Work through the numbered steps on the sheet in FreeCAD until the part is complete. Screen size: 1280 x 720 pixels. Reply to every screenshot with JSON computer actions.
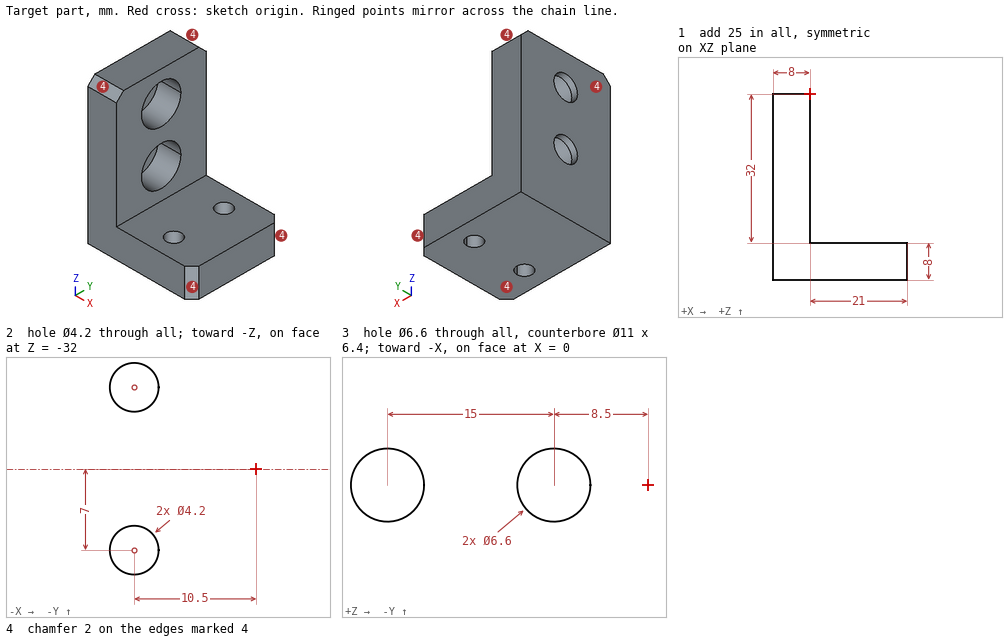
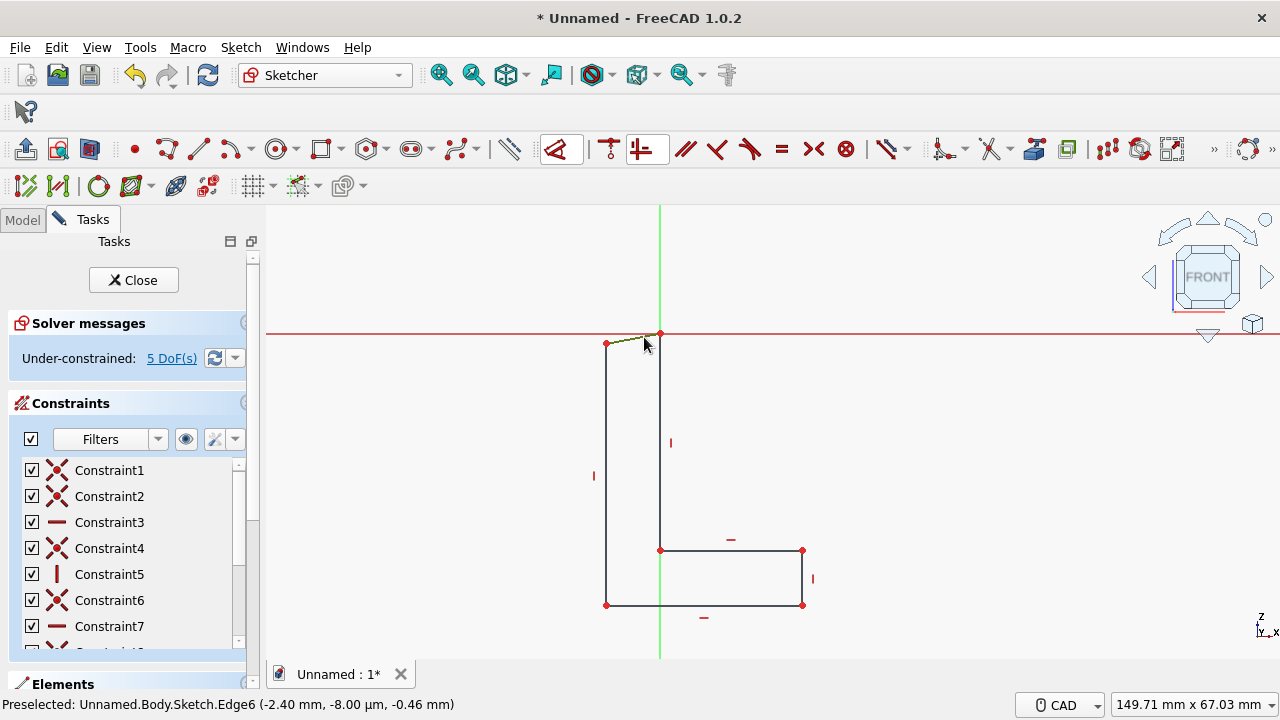
{"action": "left_click", "coordinate": [664, 150]}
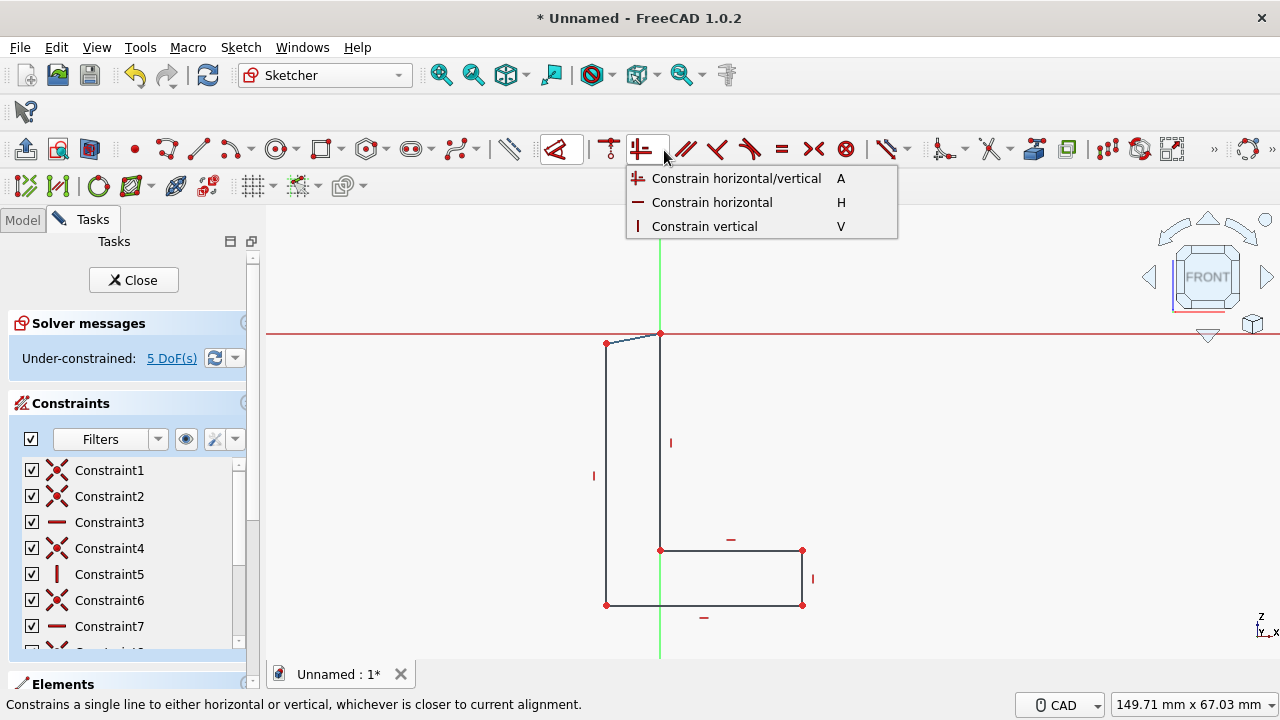
{"action": "left_click", "coordinate": [762, 202]}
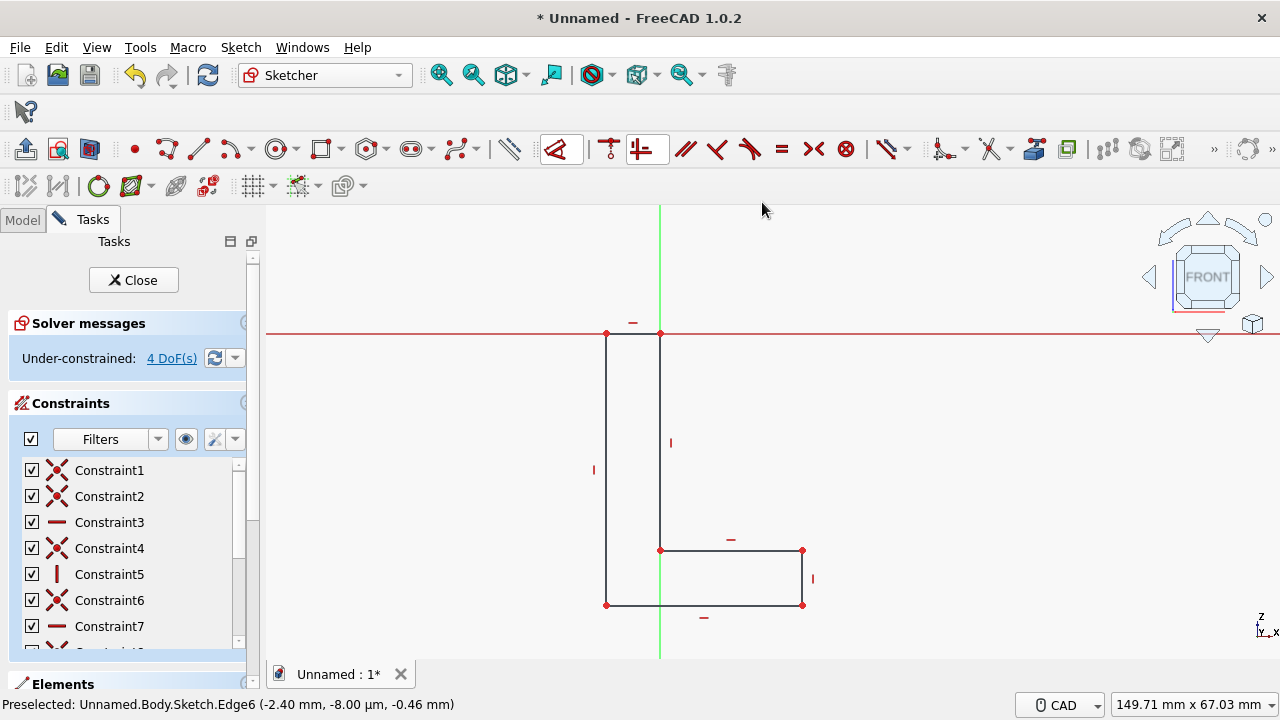
{"action": "left_click", "coordinate": [556, 150]}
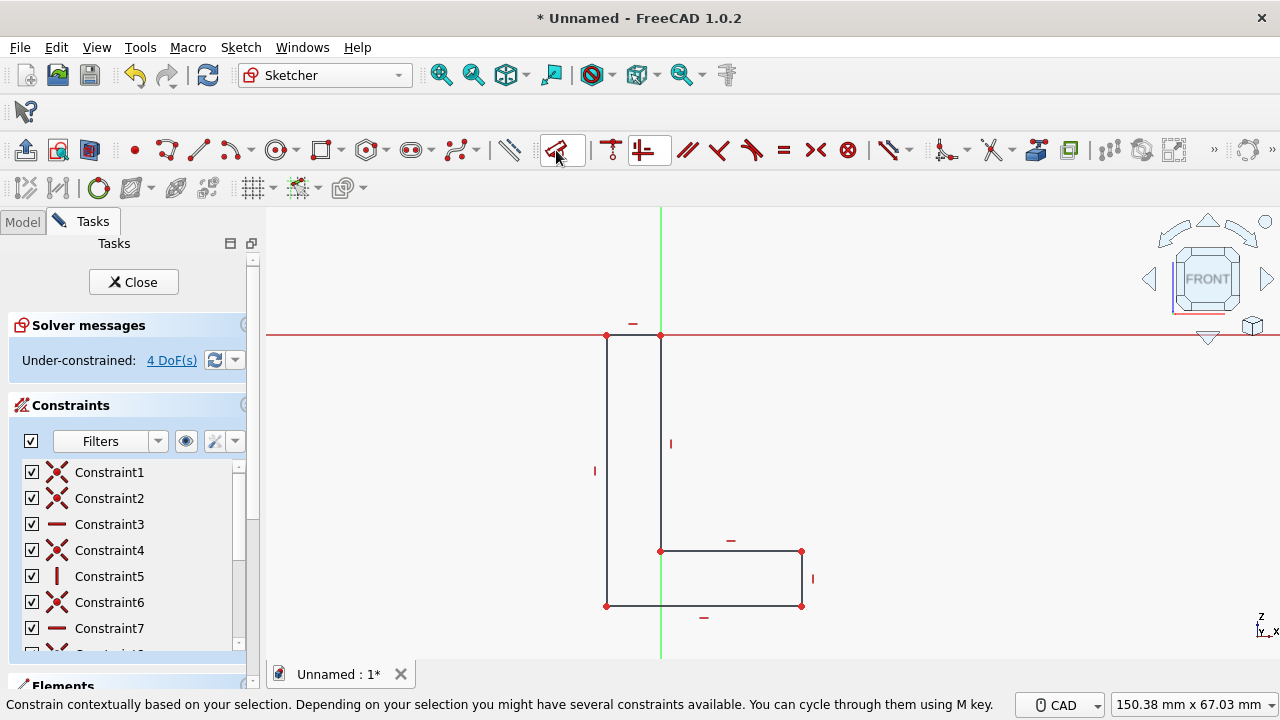
{"action": "left_click", "coordinate": [802, 568]}
{"action": "left_click", "coordinate": [836, 579]}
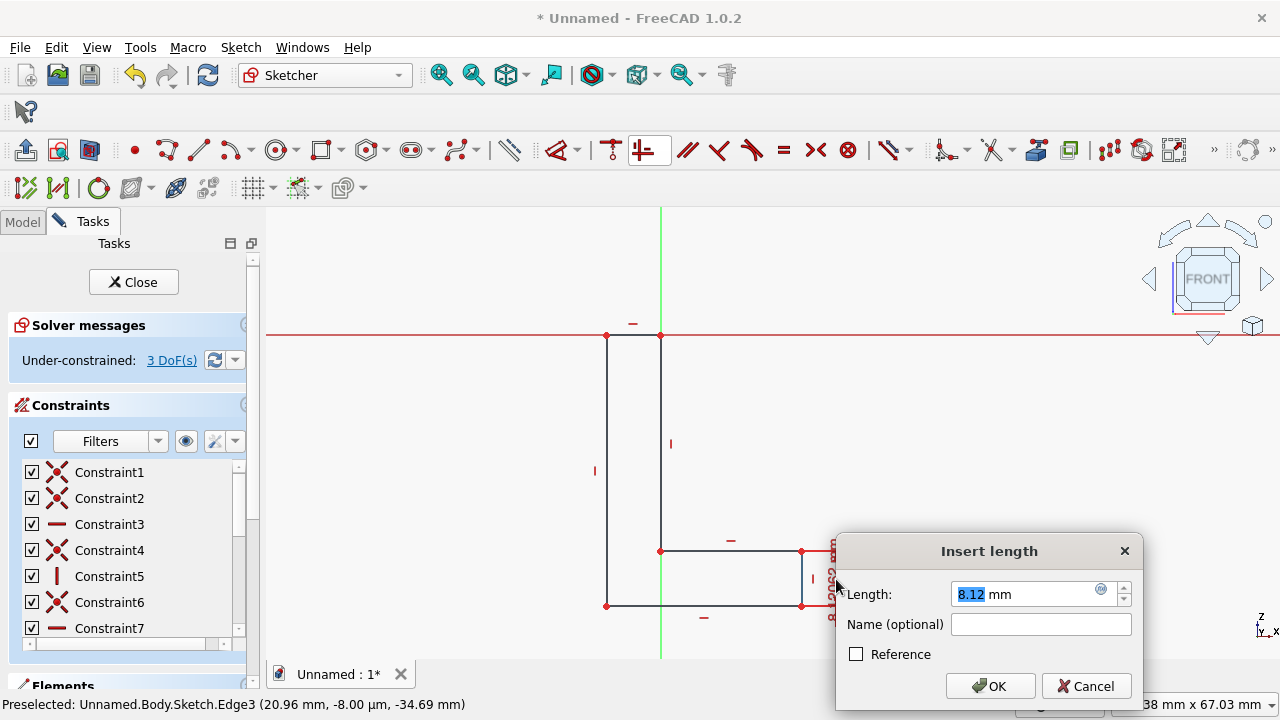
{"action": "type", "text": "8"}
{"action": "key", "text": "Return"}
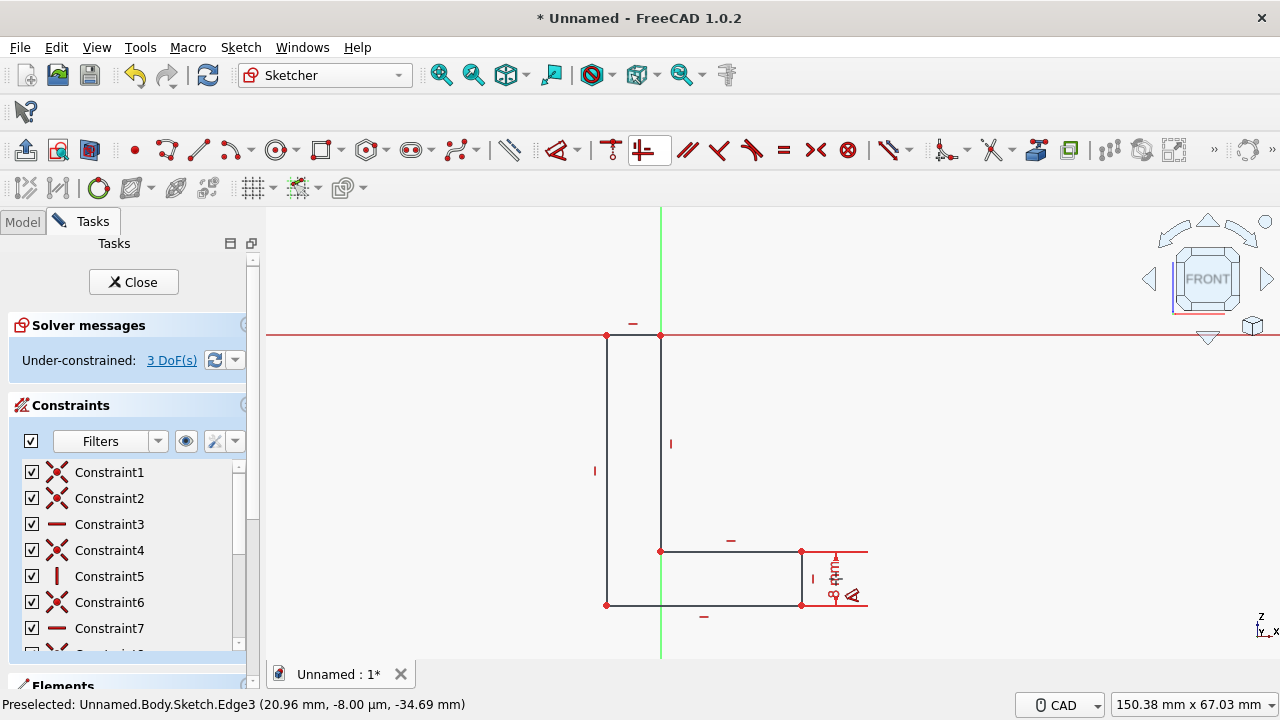
{"action": "left_click", "coordinate": [623, 335]}
{"action": "left_click", "coordinate": [634, 301]}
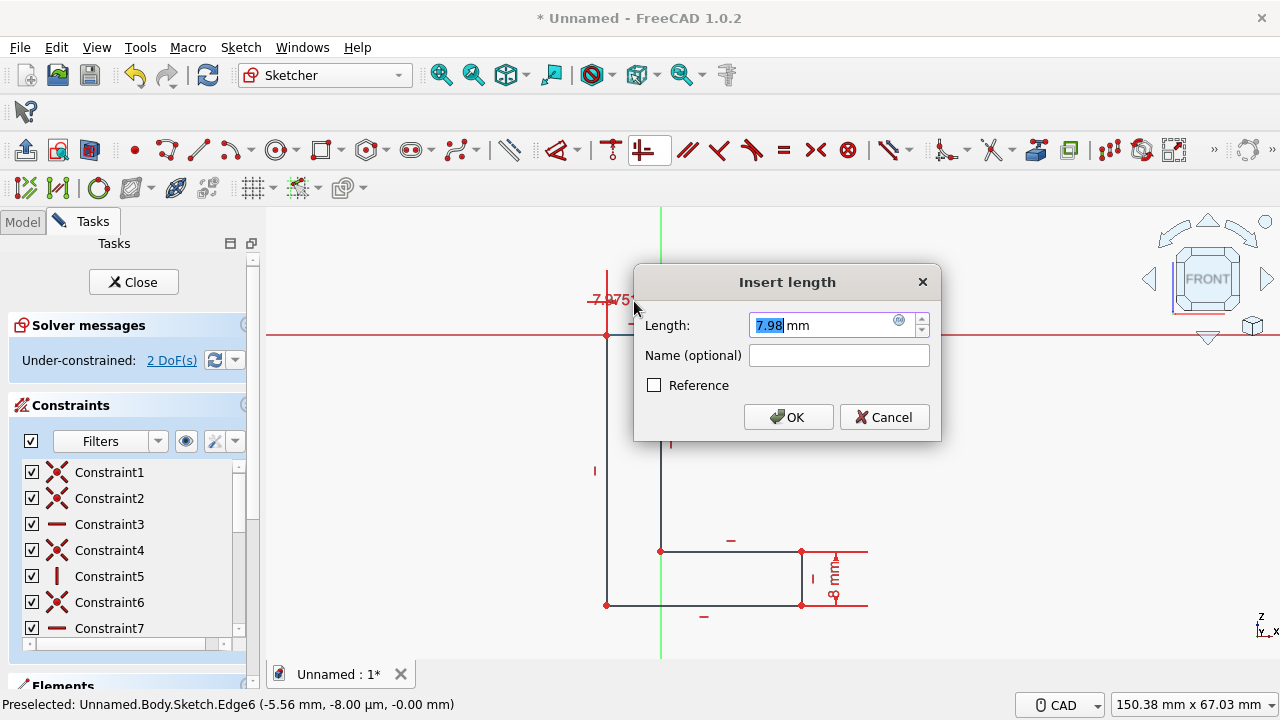
{"action": "type", "text": "8"}
{"action": "key", "text": "Return"}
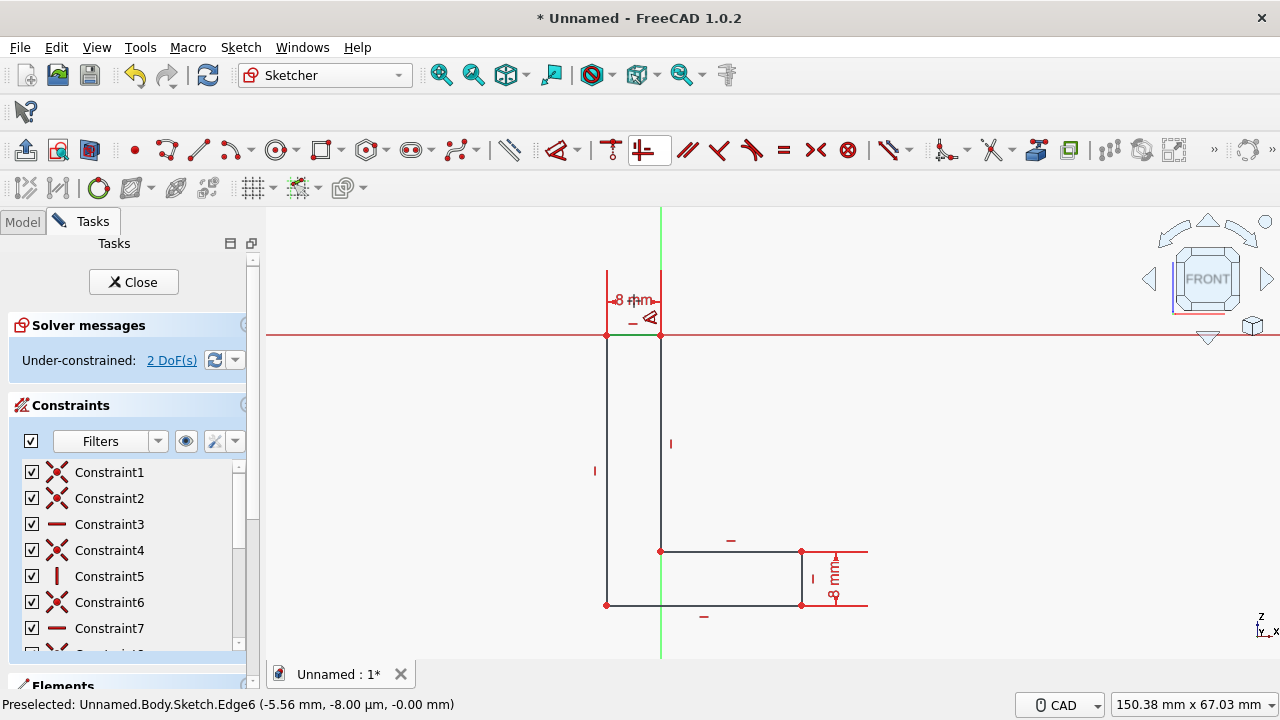
{"action": "left_click", "coordinate": [661, 400]}
{"action": "left_click", "coordinate": [627, 443]}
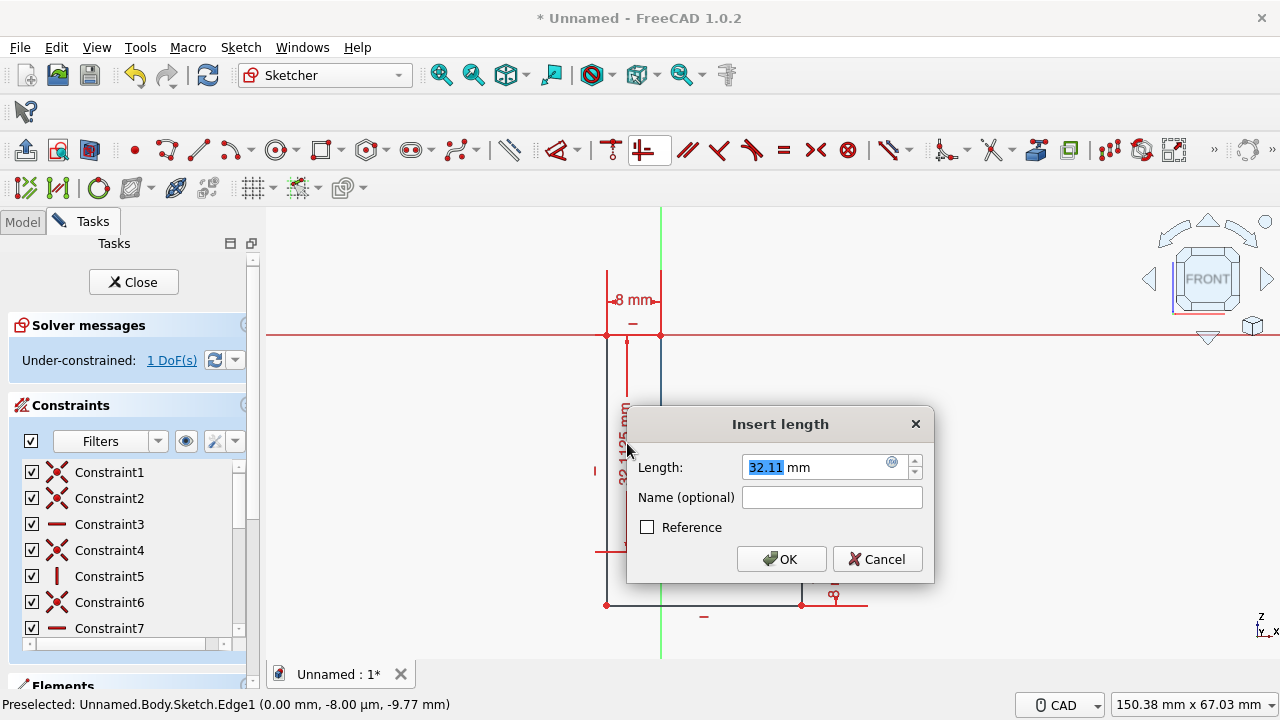
{"action": "type", "text": "32"}
{"action": "key", "text": "Return"}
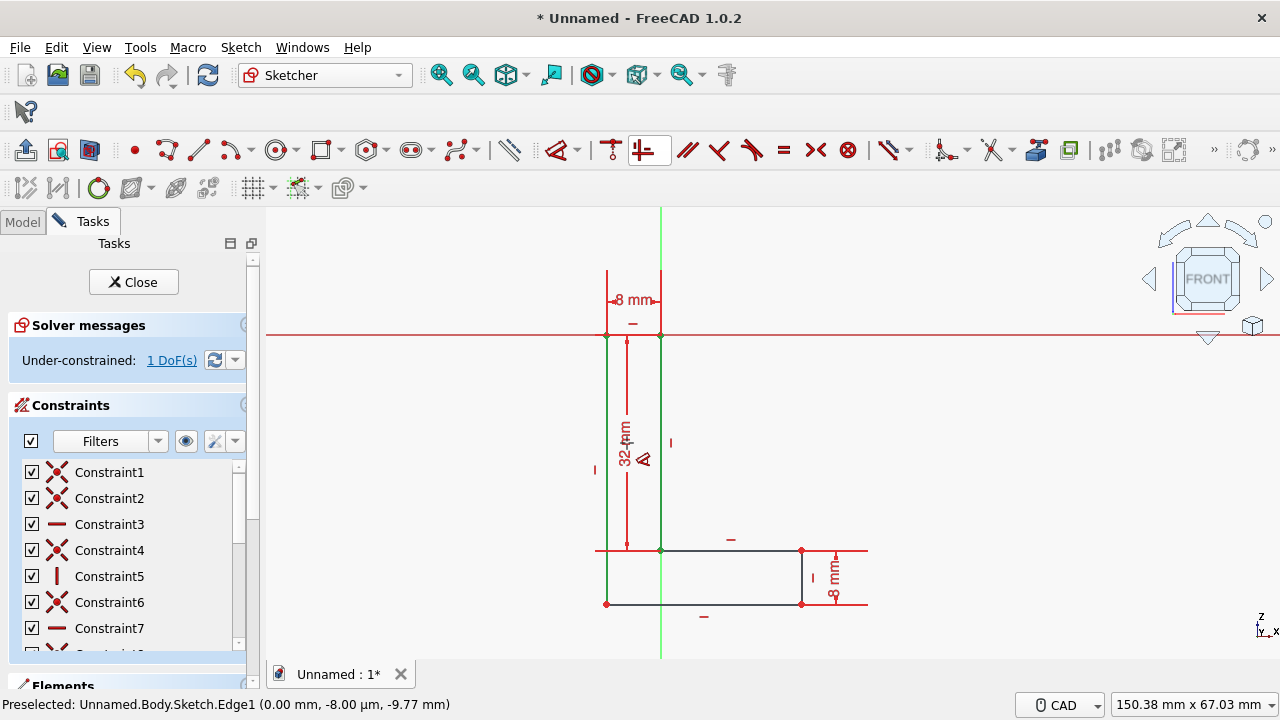
{"action": "left_click", "coordinate": [703, 551]}
{"action": "left_click", "coordinate": [731, 585]}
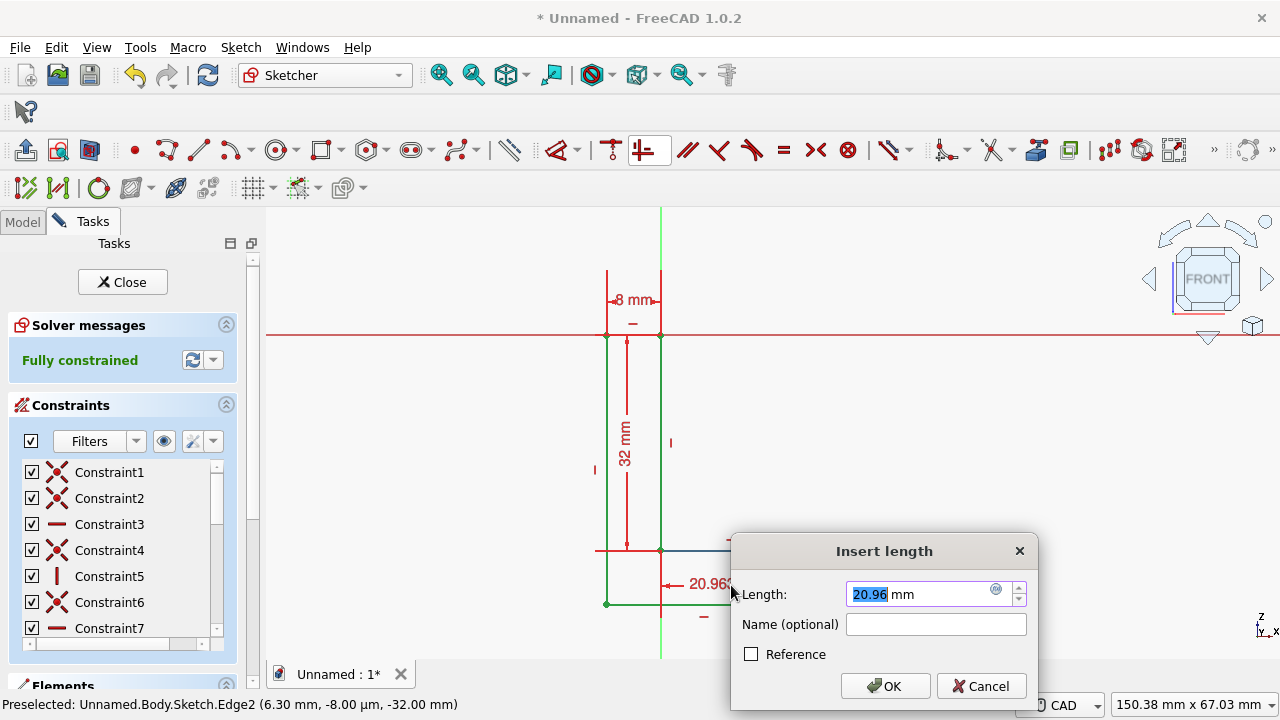
{"action": "type", "text": "21"}
{"action": "key", "text": "Return"}
{"action": "key", "text": "Escape"}